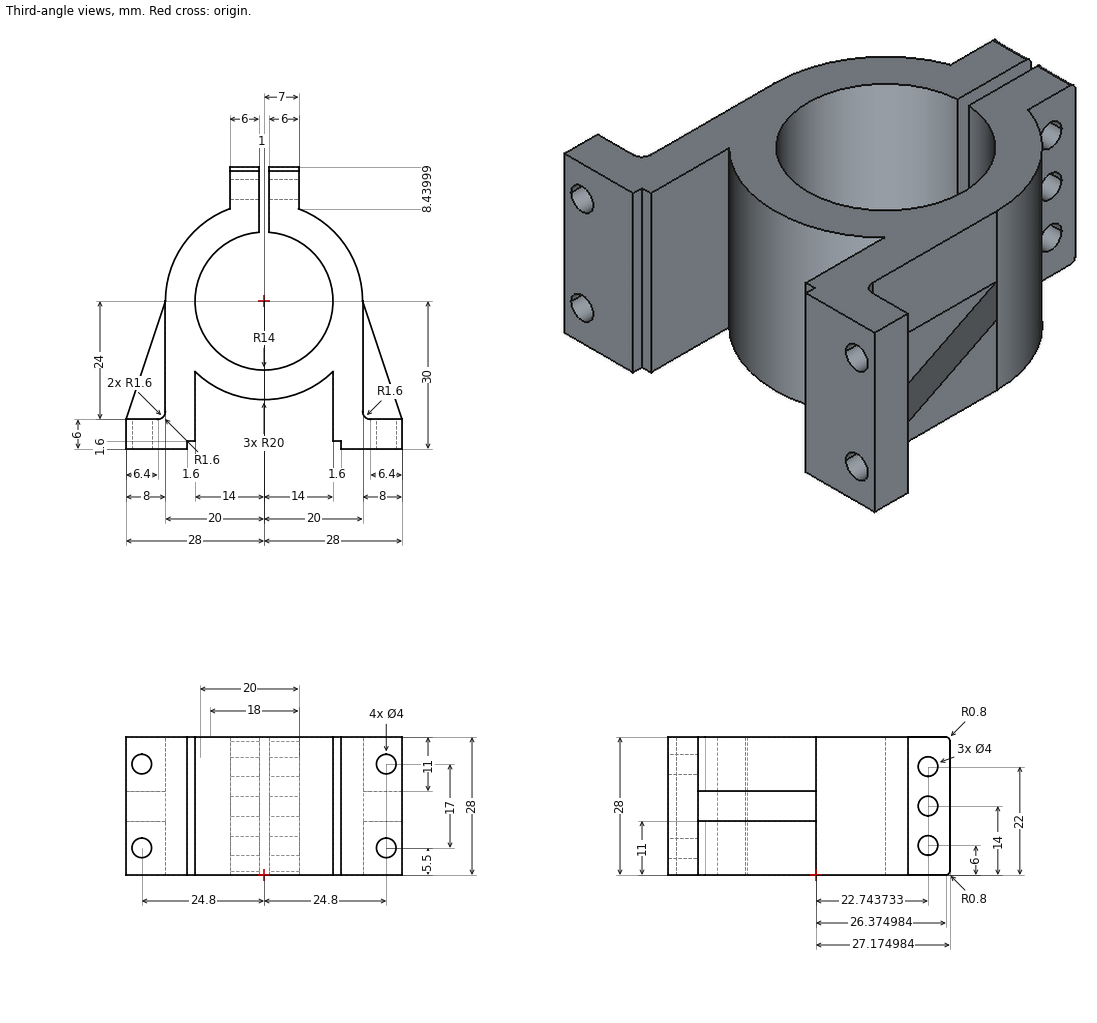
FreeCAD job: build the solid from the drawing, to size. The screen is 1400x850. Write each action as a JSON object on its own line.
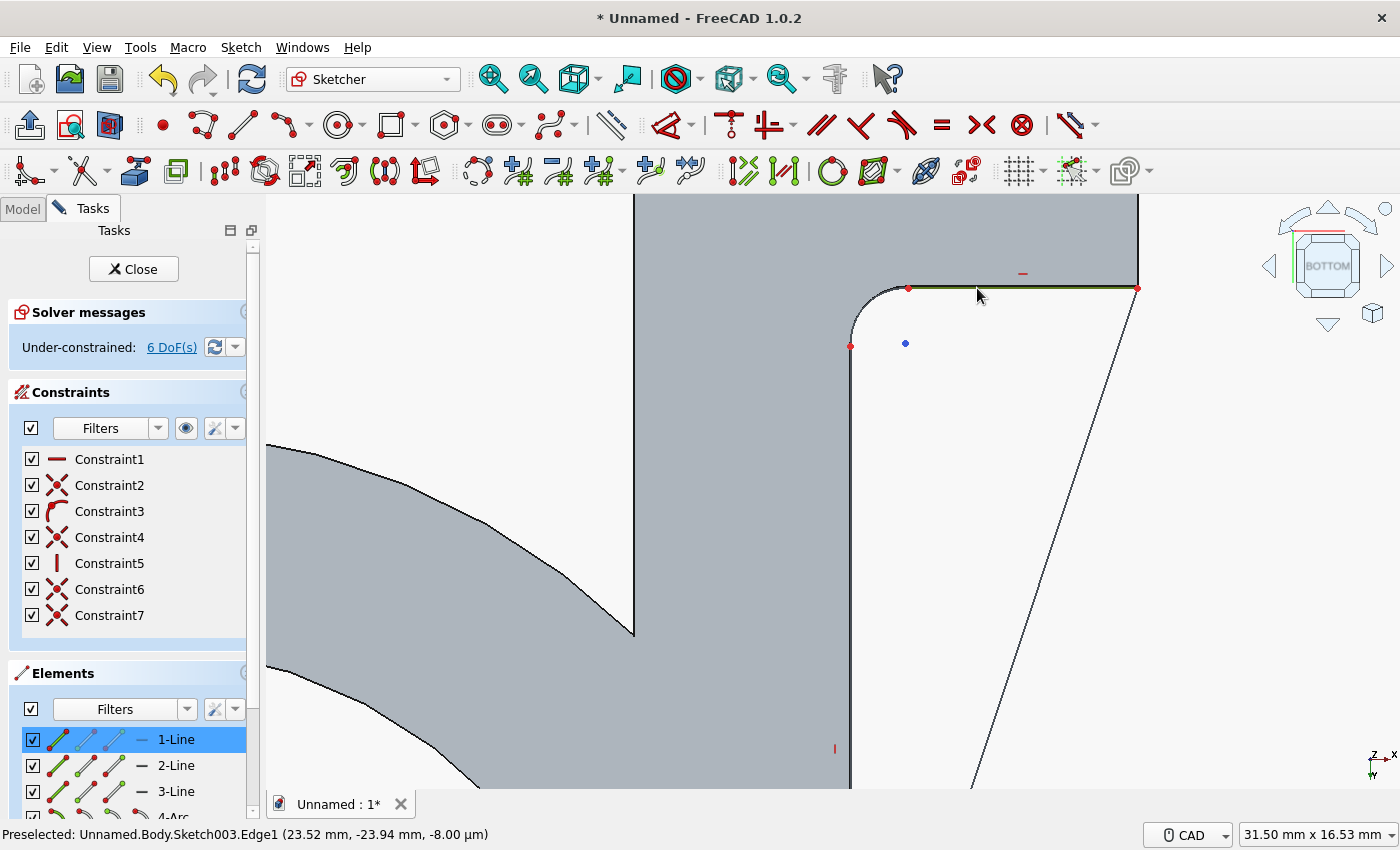
{"action": "left_click", "coordinate": [882, 294]}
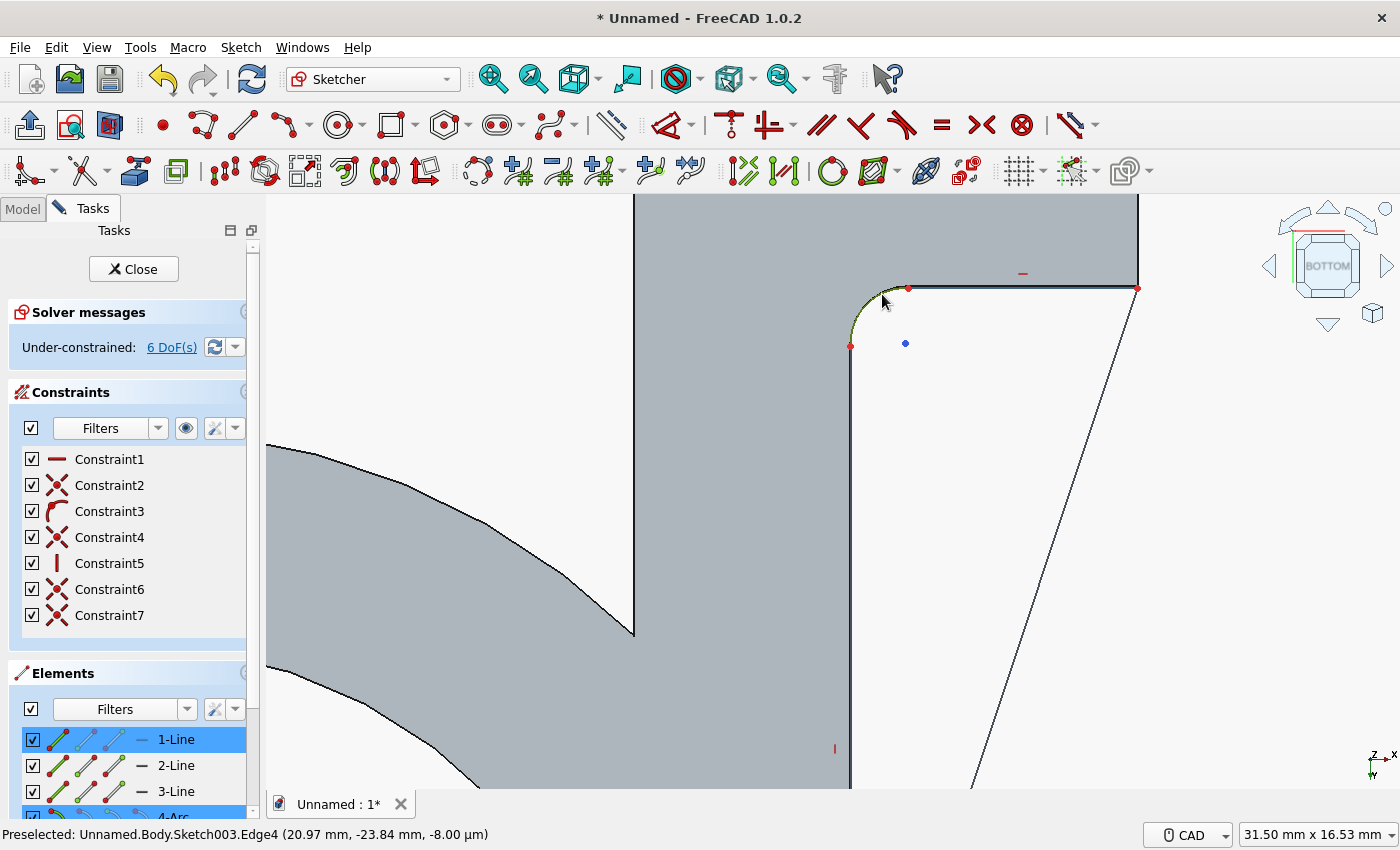
{"action": "left_click", "coordinate": [902, 126]}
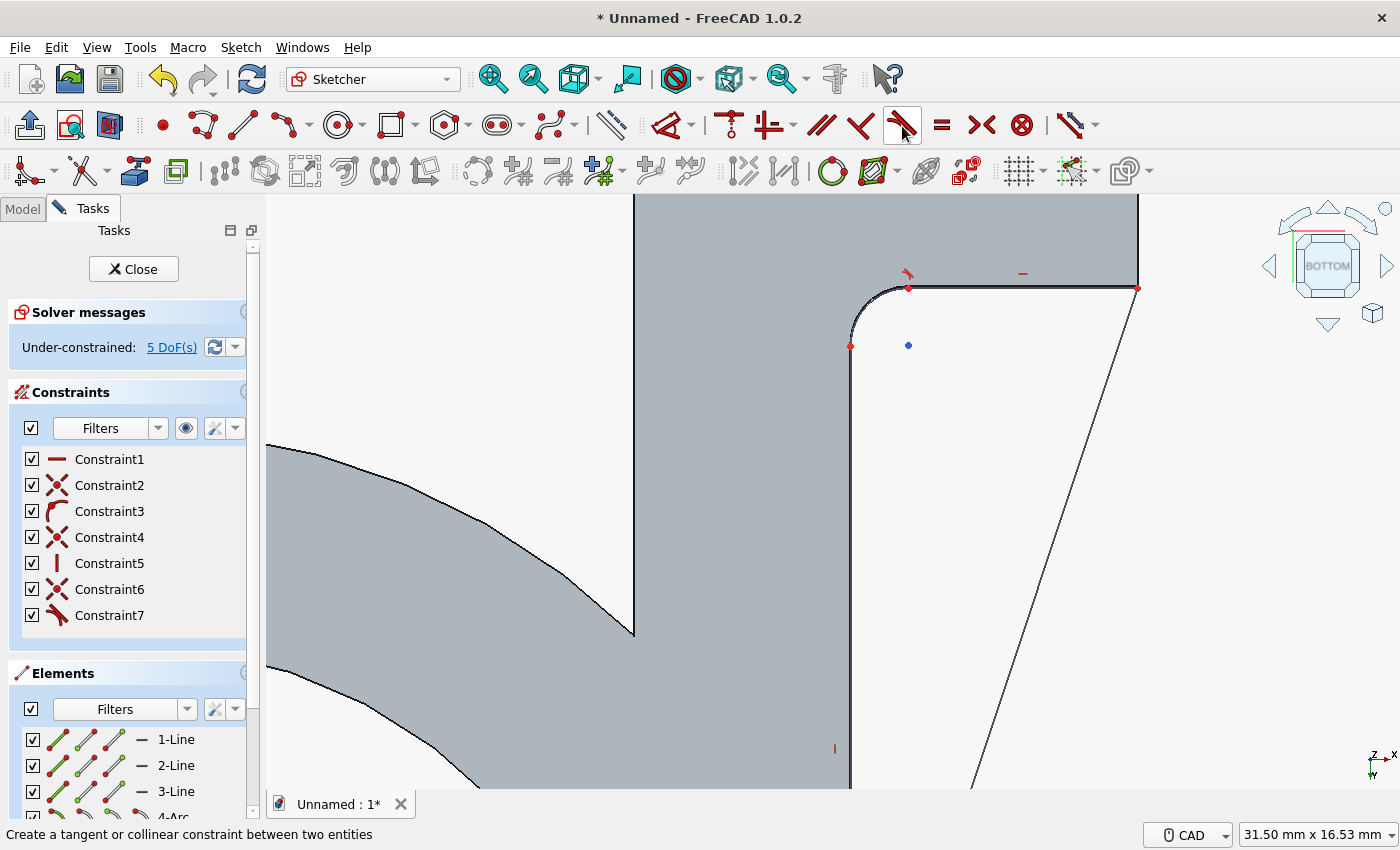
{"action": "left_click", "coordinate": [851, 587]}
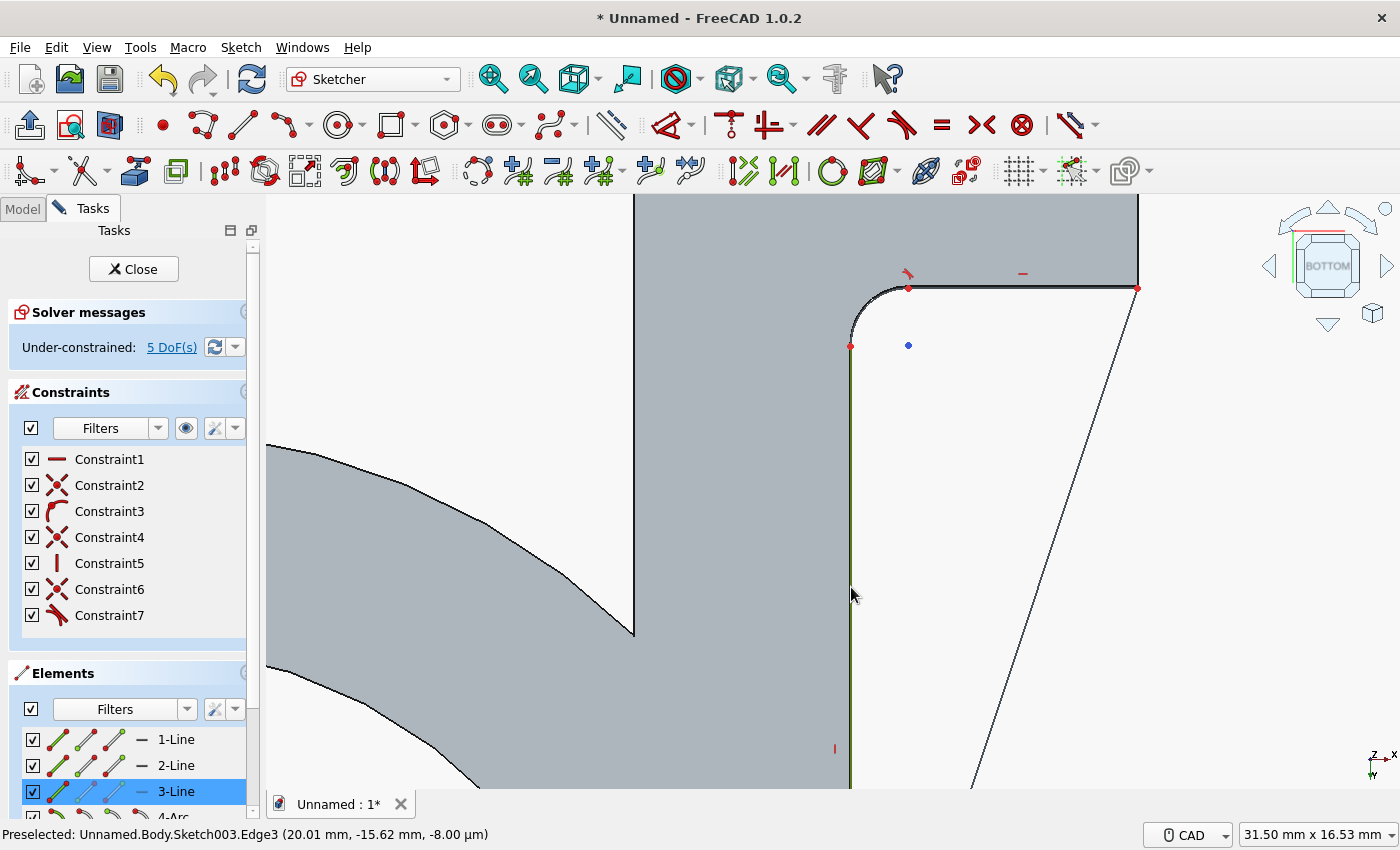
{"action": "left_click", "coordinate": [882, 294]}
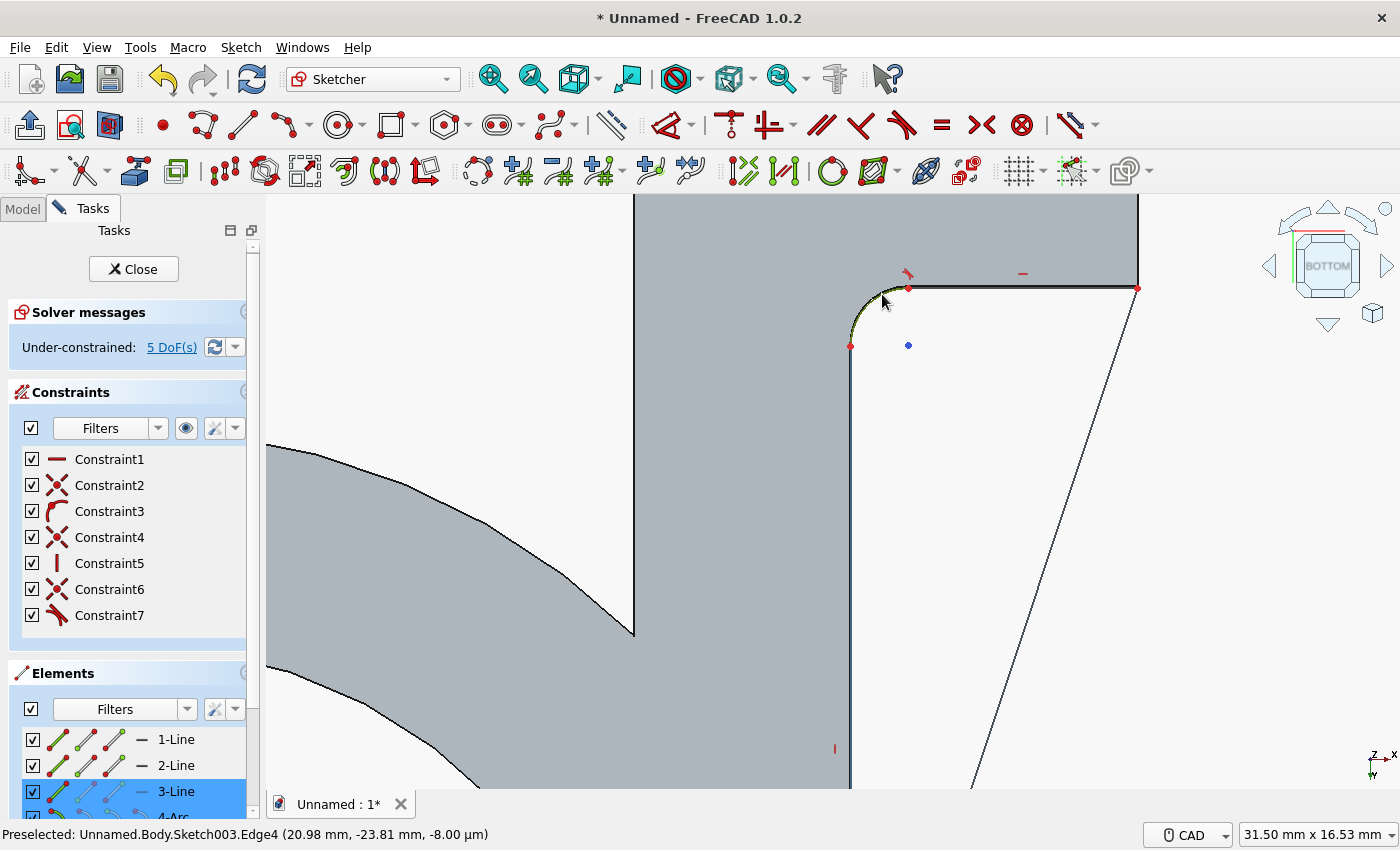
{"action": "left_click", "coordinate": [902, 126]}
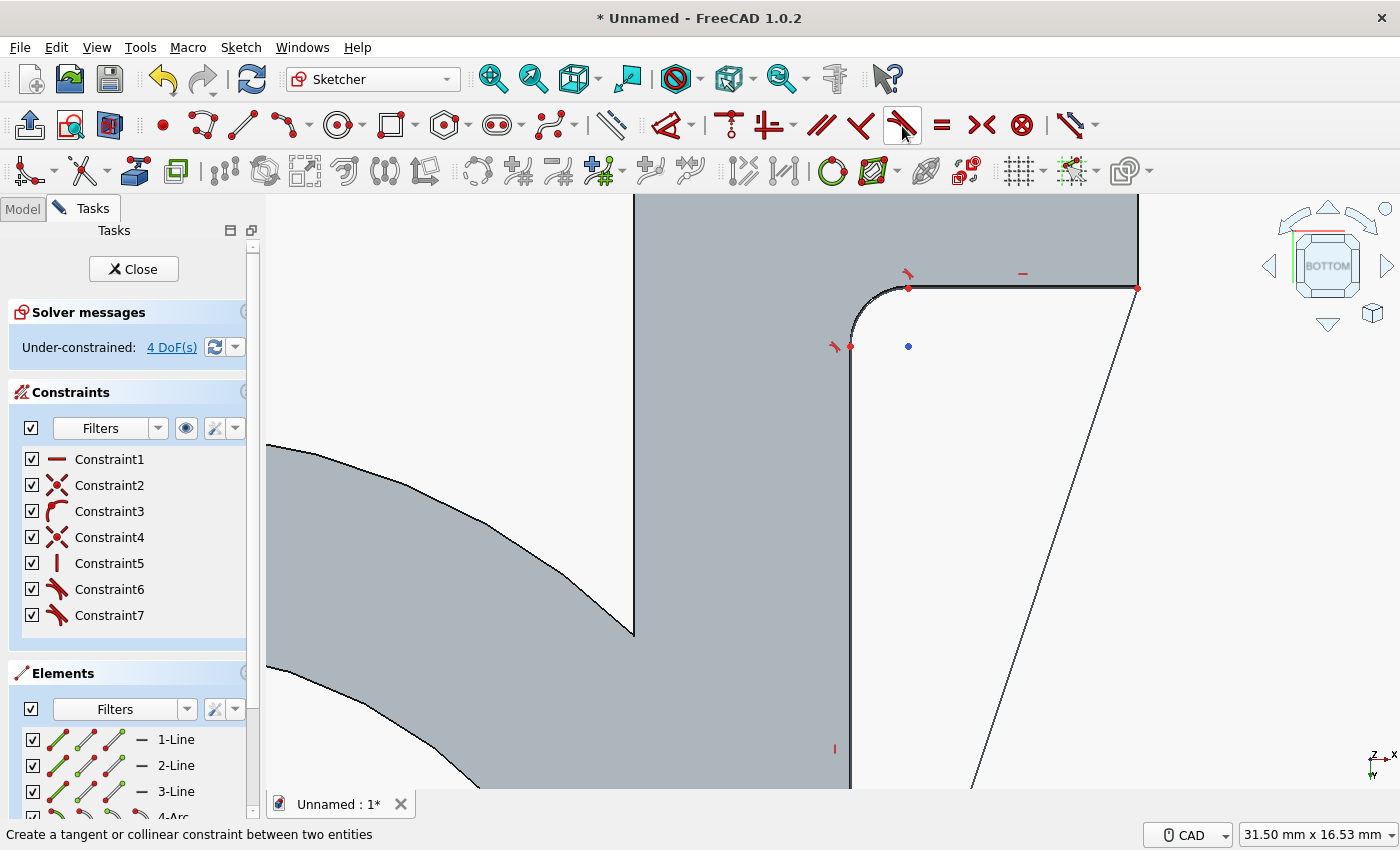
{"action": "left_click", "coordinate": [666, 126]}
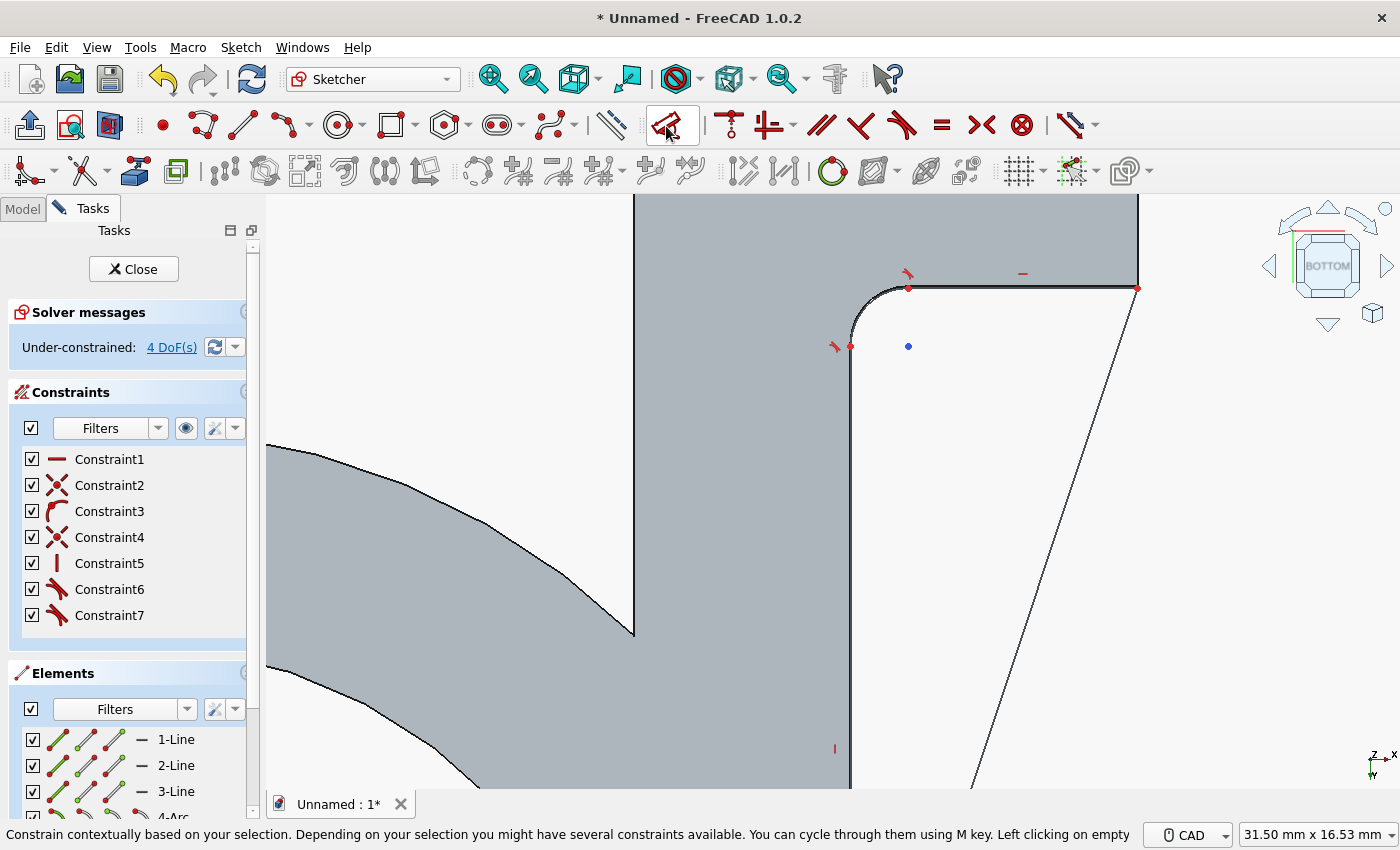
{"action": "left_click", "coordinate": [882, 294]}
{"action": "left_click", "coordinate": [867, 266]}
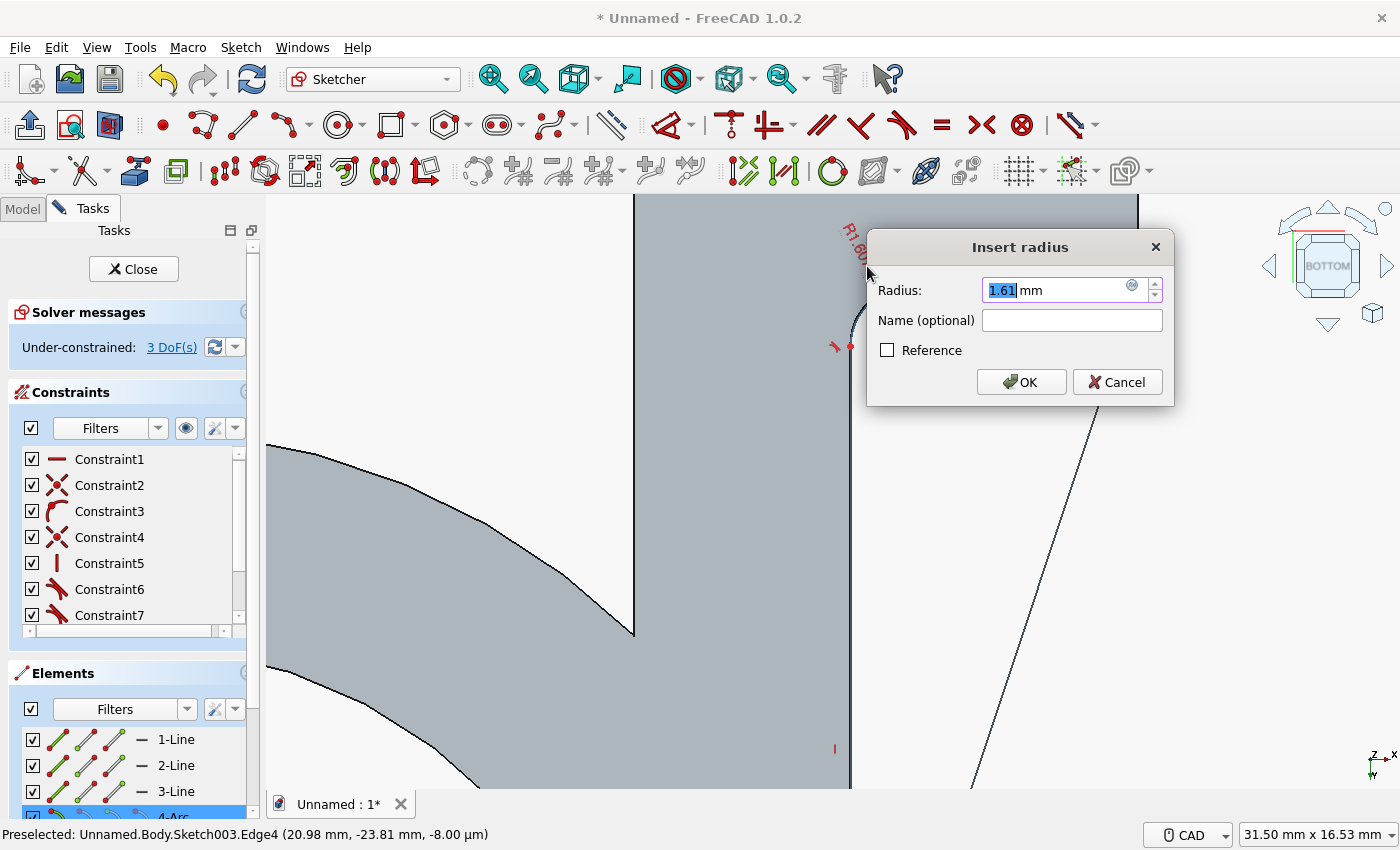
{"action": "type", "text": "1.6"}
{"action": "key", "text": "Return"}